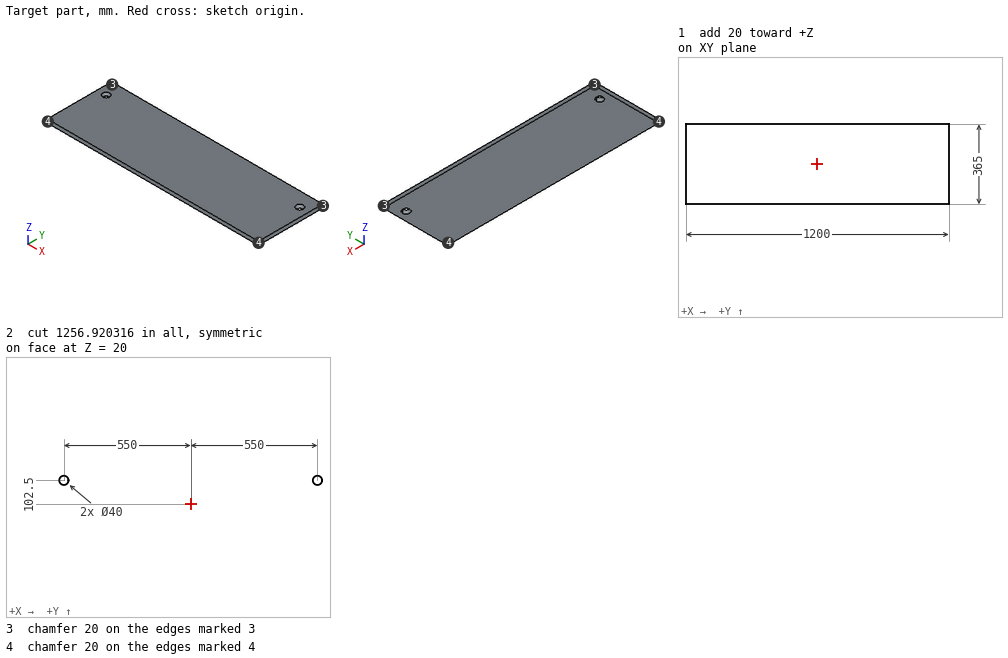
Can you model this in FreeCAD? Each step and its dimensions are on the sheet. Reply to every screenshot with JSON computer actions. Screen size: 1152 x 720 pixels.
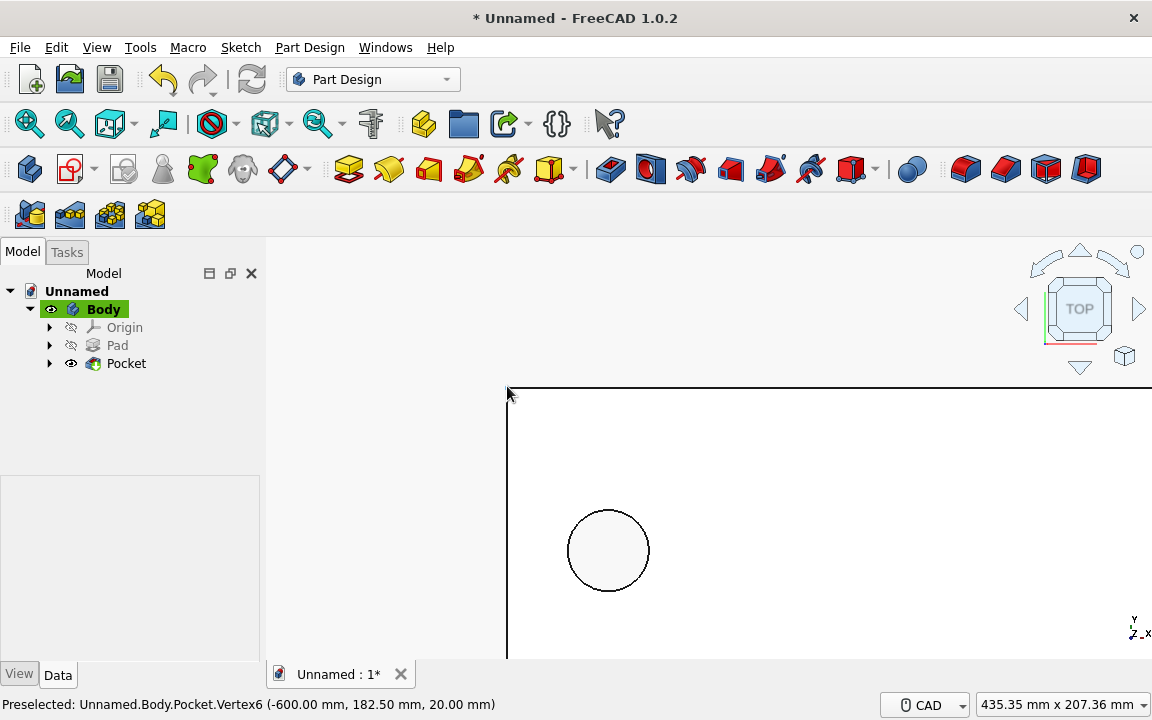
{"action": "key", "text": "v f"}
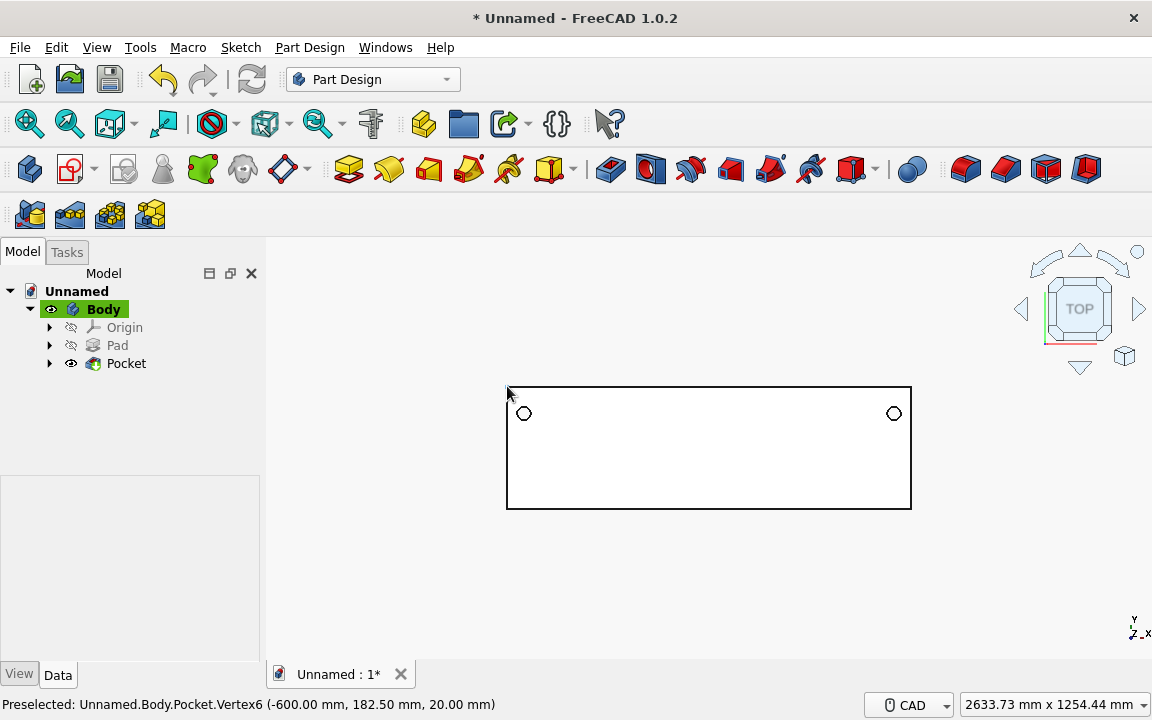
{"action": "key", "text": "1"}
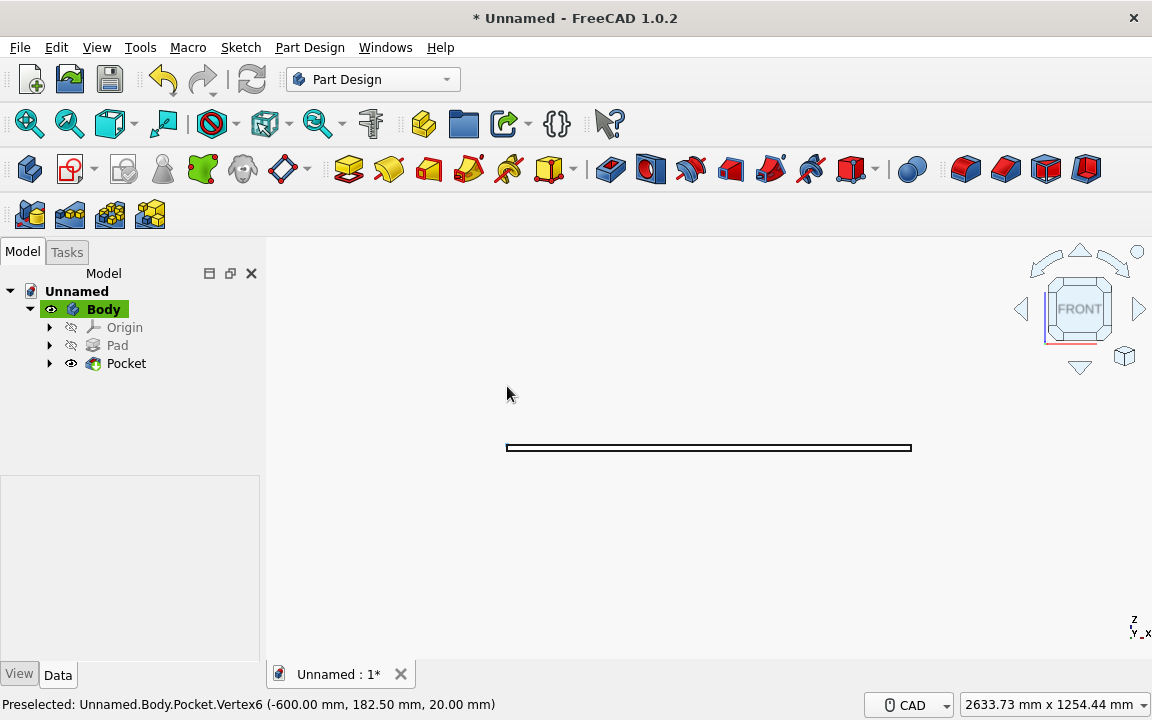
{"action": "scroll", "coordinate": [507, 447], "scroll_direction": "up", "scroll_amount": 9}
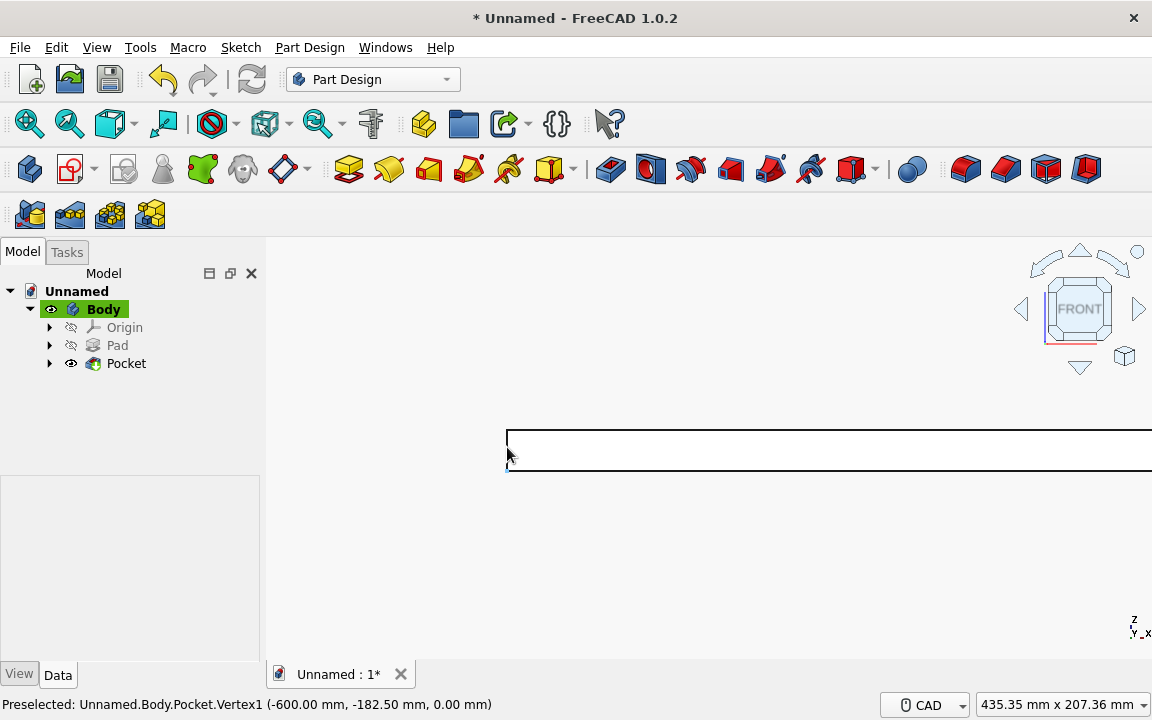
{"action": "left_click", "coordinate": [30, 124]}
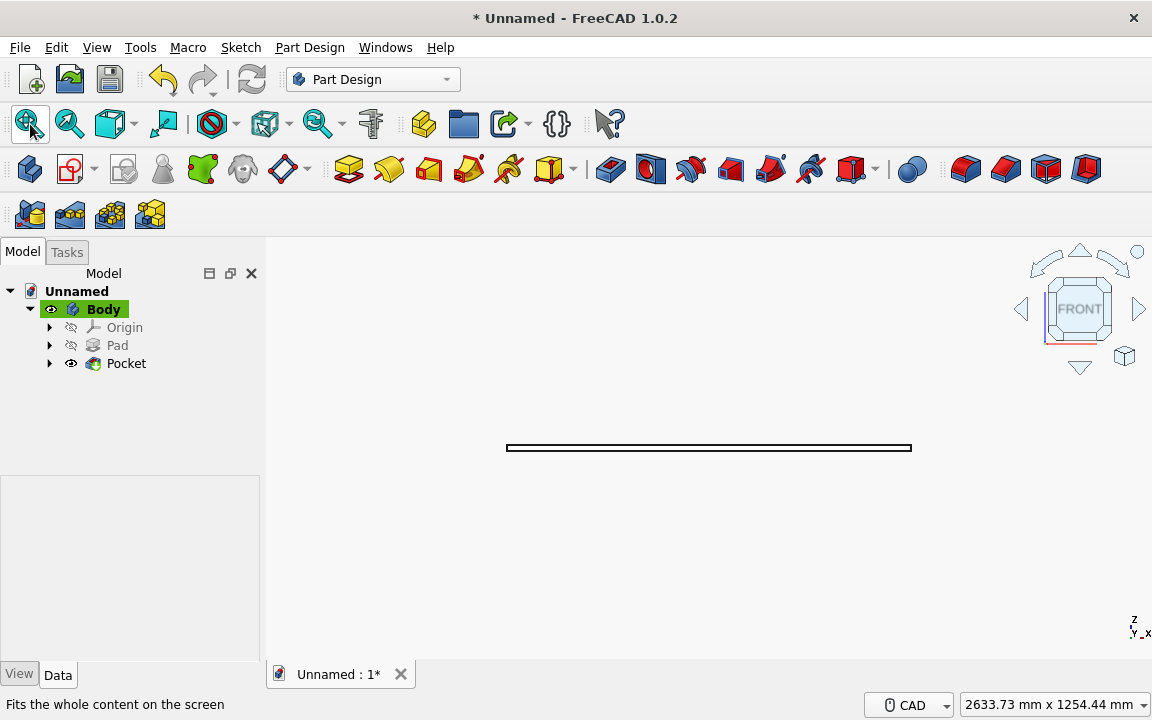
{"action": "key", "text": "3"}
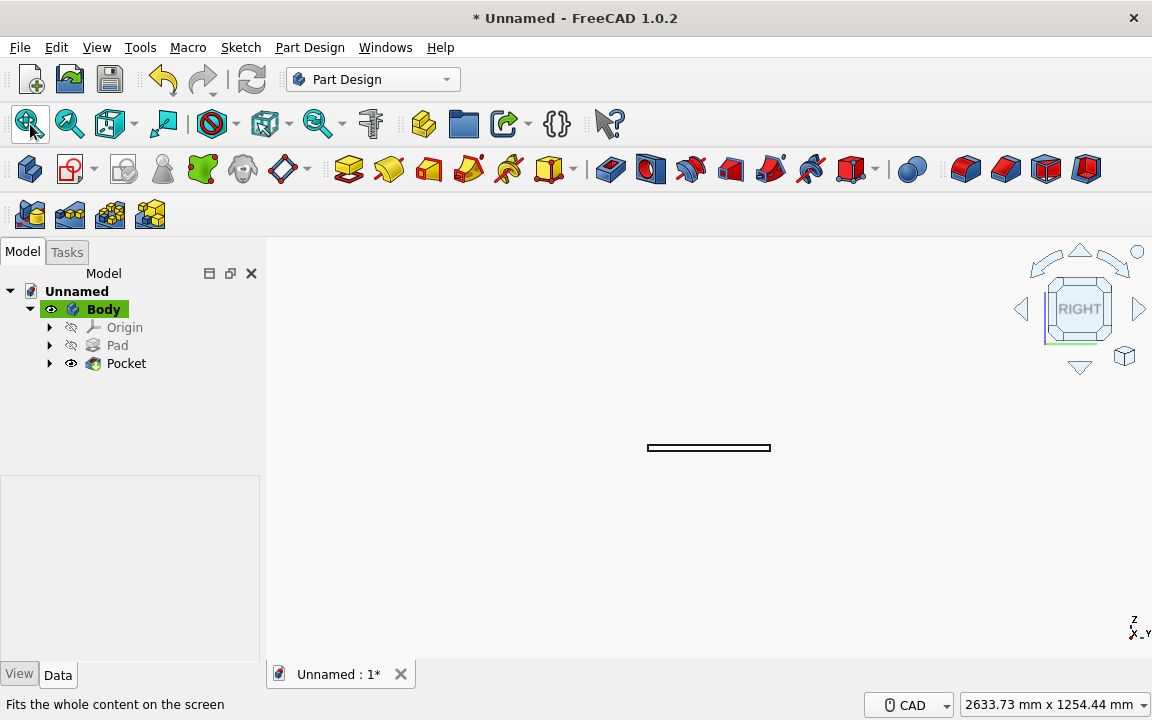
{"action": "key", "text": "v f"}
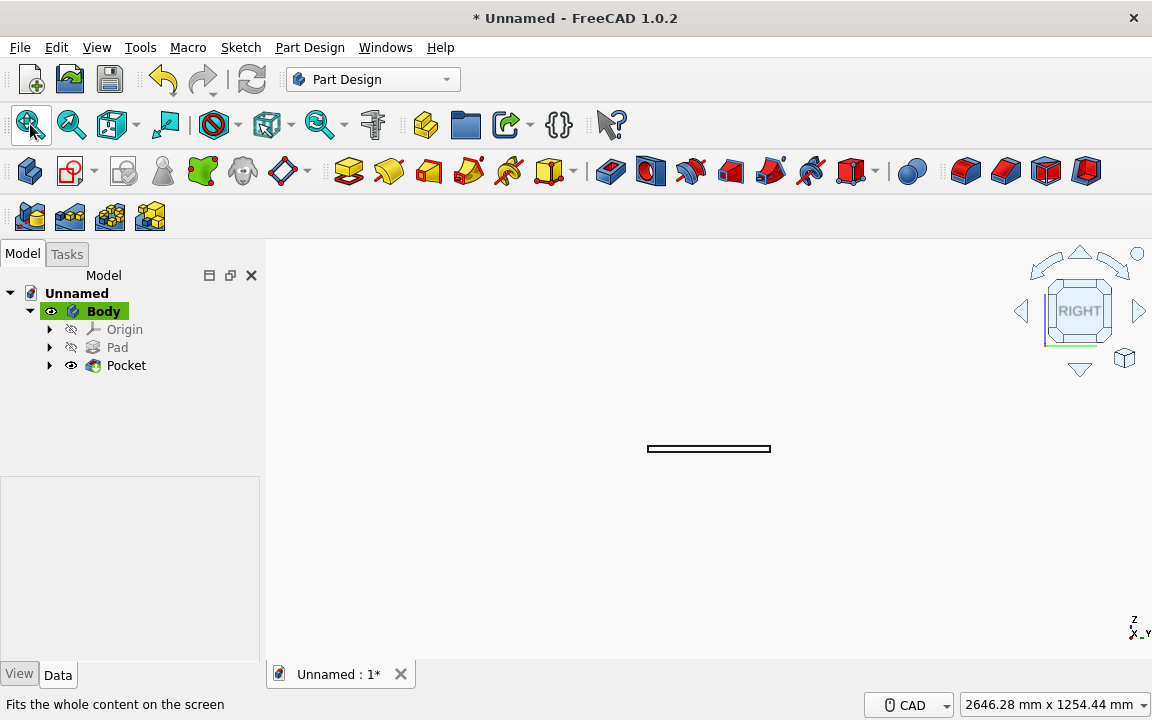
{"action": "scroll", "coordinate": [770, 448], "scroll_direction": "up", "scroll_amount": 9}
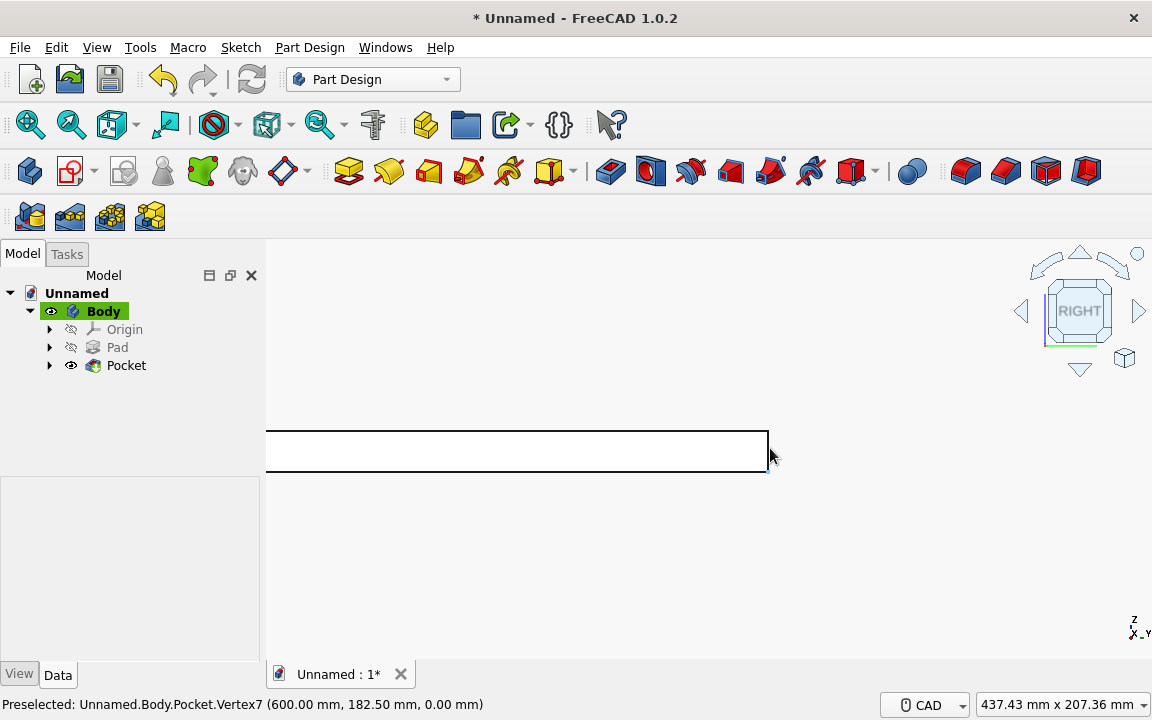
{"action": "left_click", "coordinate": [768, 451]}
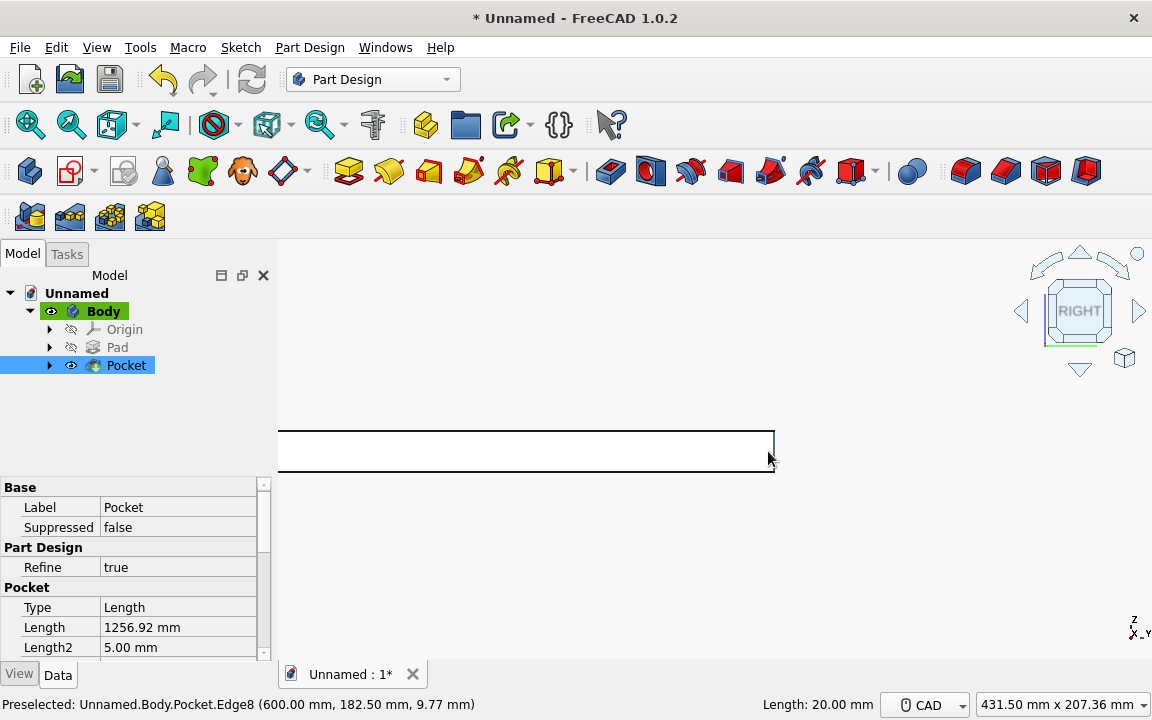
{"action": "key", "text": "v f"}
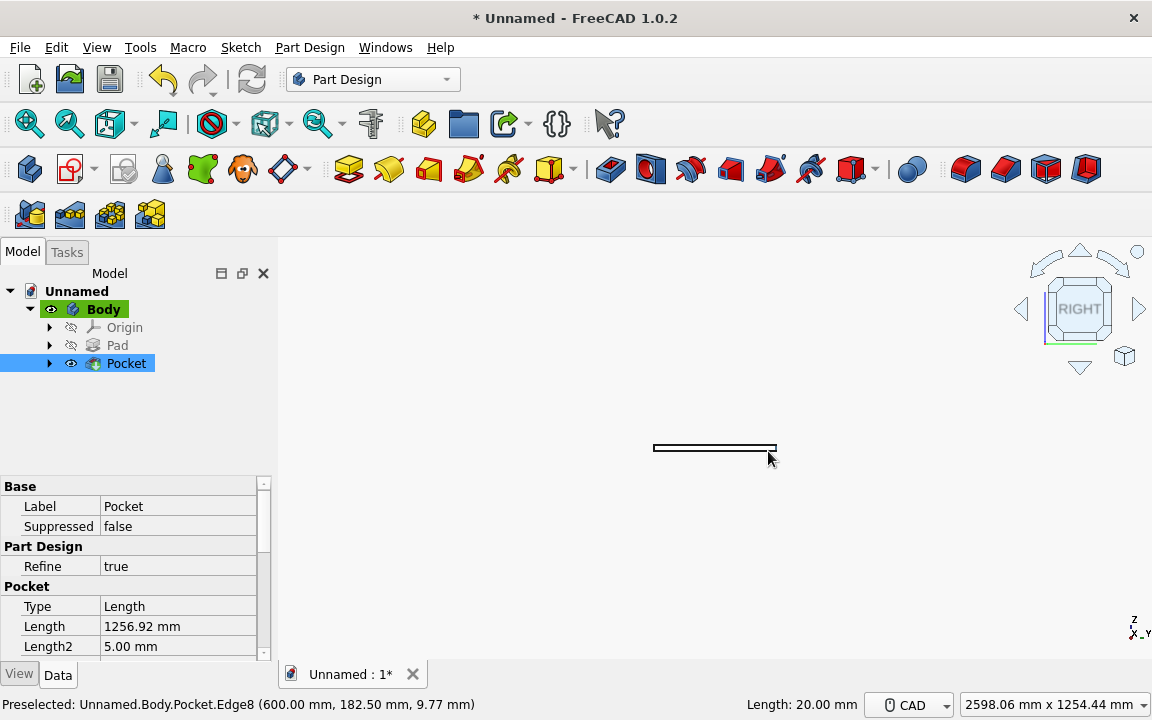
{"action": "key", "text": "5"}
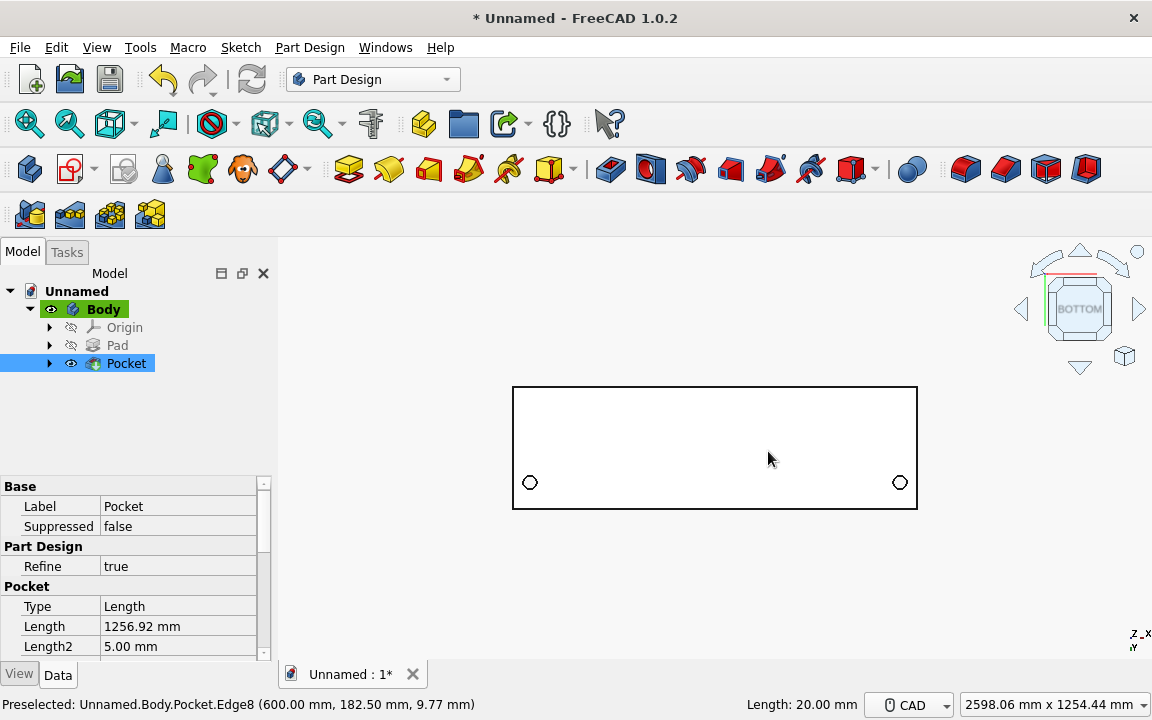
{"action": "scroll", "coordinate": [513, 508], "scroll_direction": "up", "scroll_amount": 9}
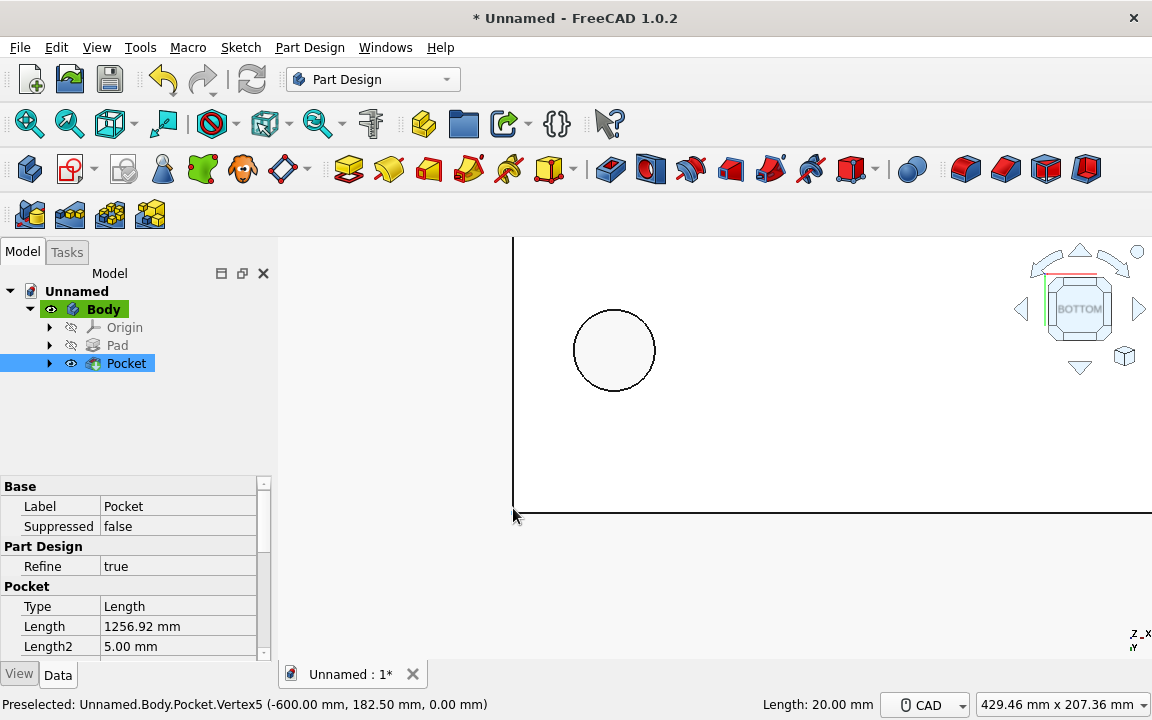
{"action": "left_click", "coordinate": [30, 124]}